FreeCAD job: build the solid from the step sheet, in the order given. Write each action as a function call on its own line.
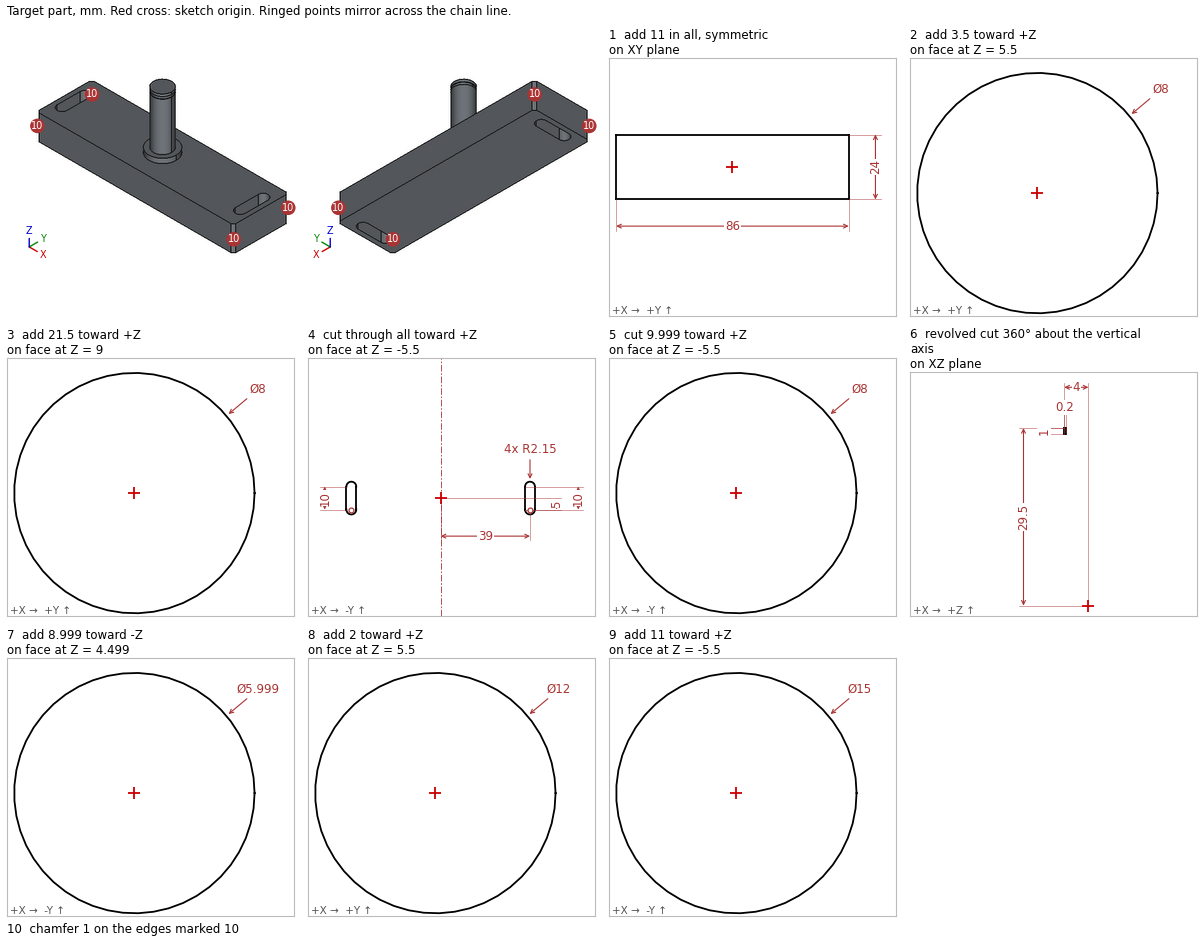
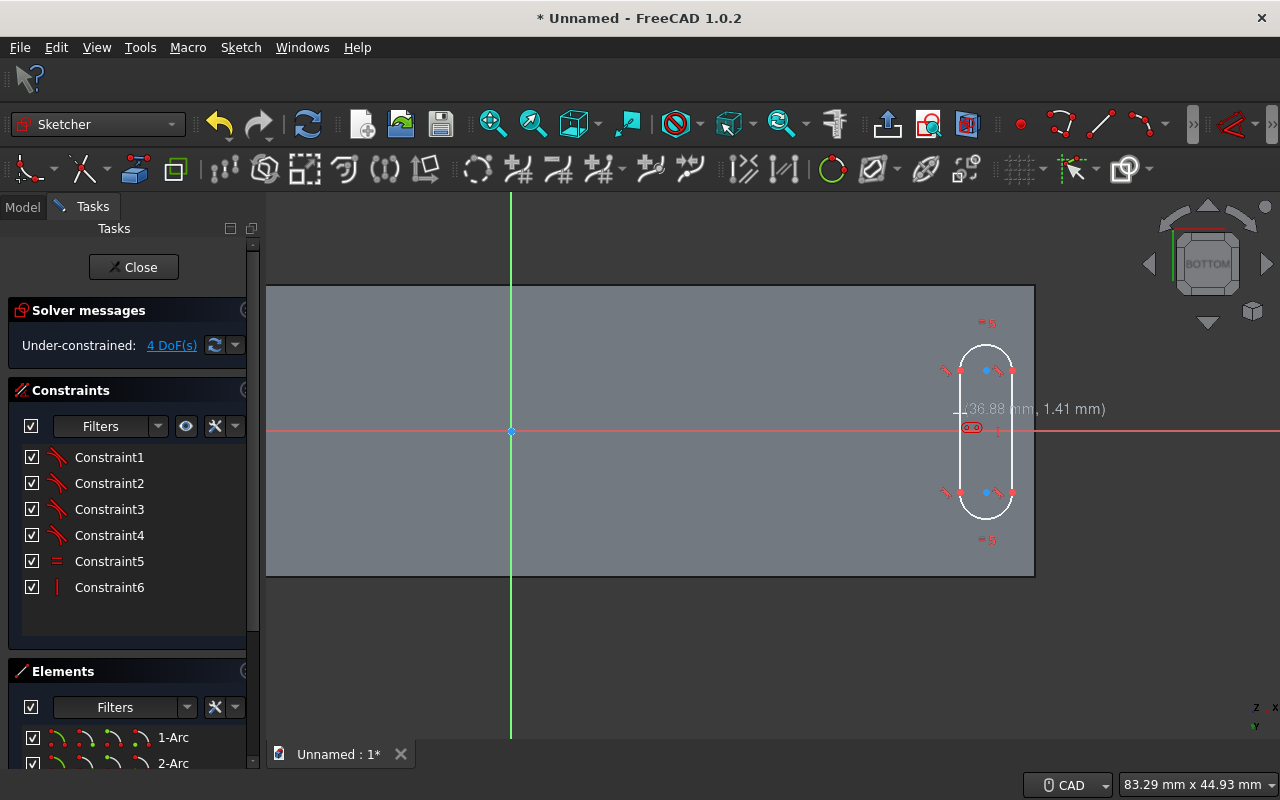
scroll(940, 507, down, 3)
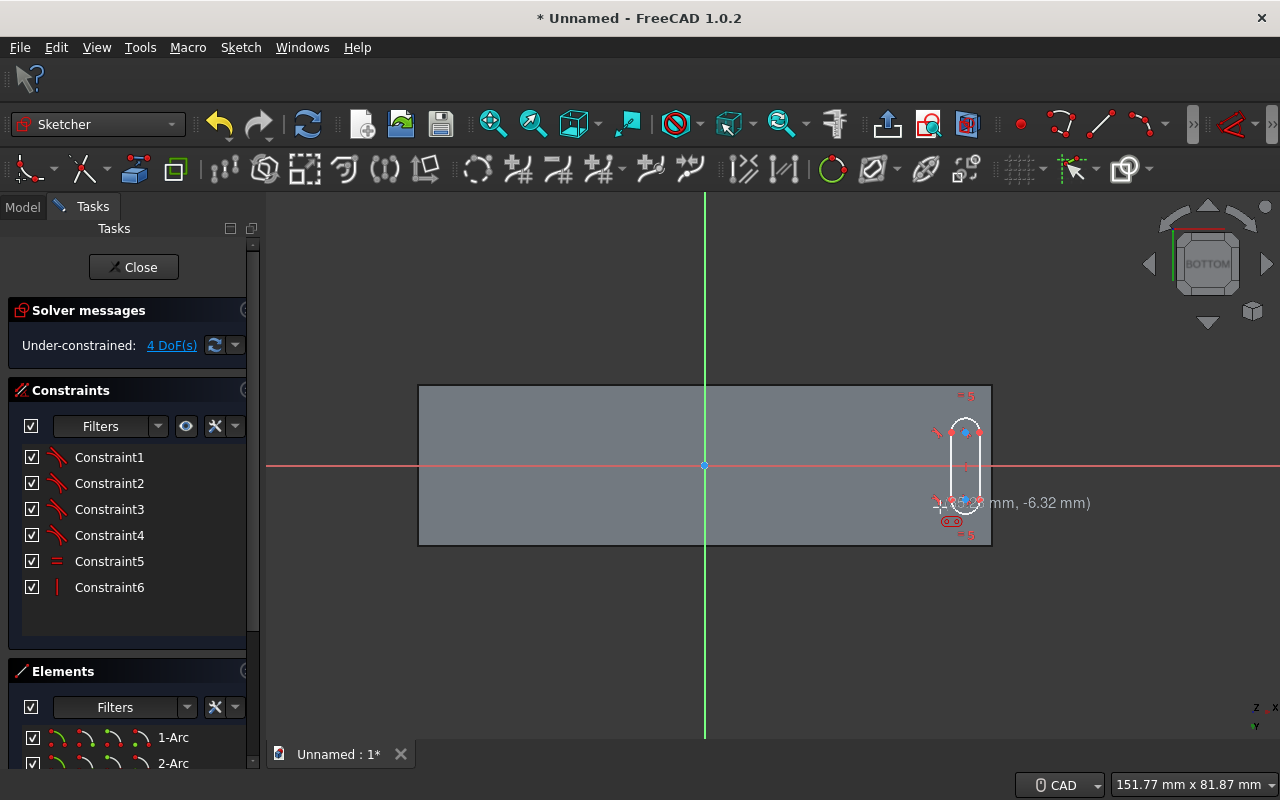
scroll(444, 499, up, 3)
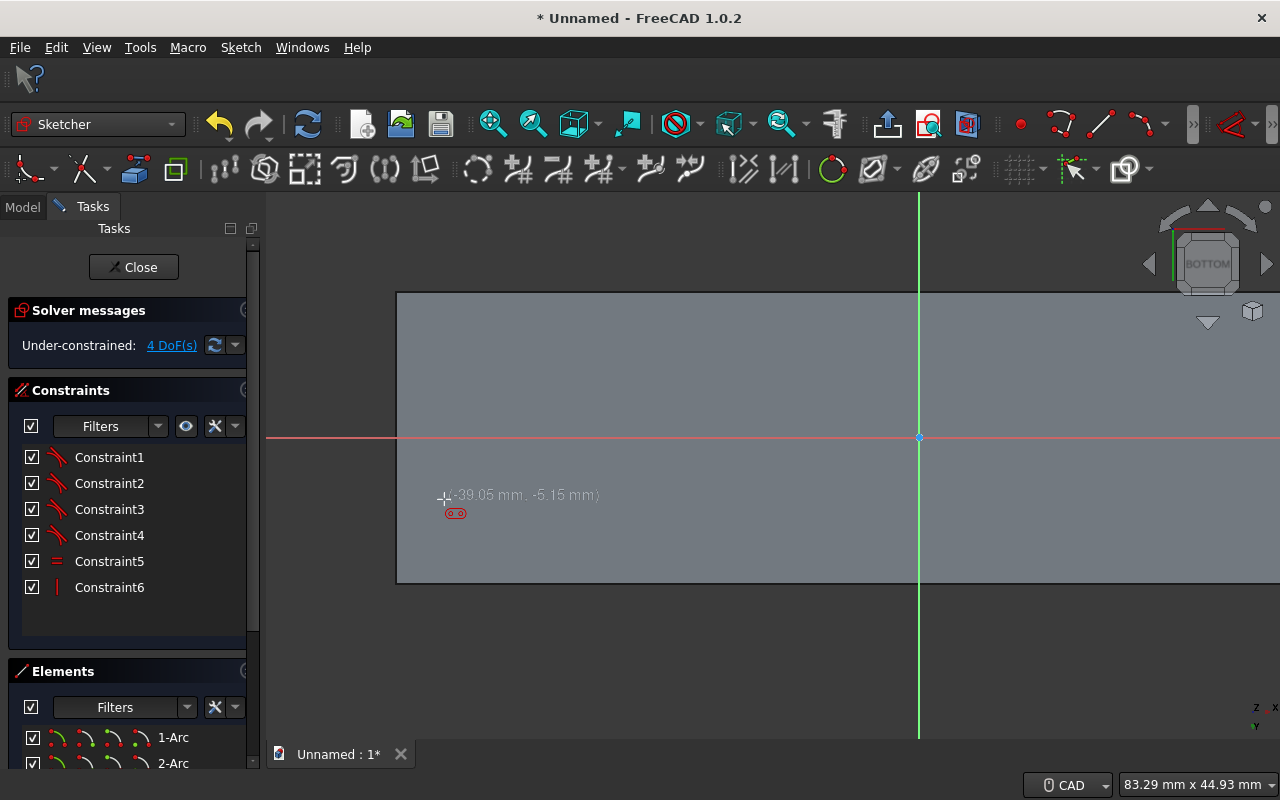
click(444, 499)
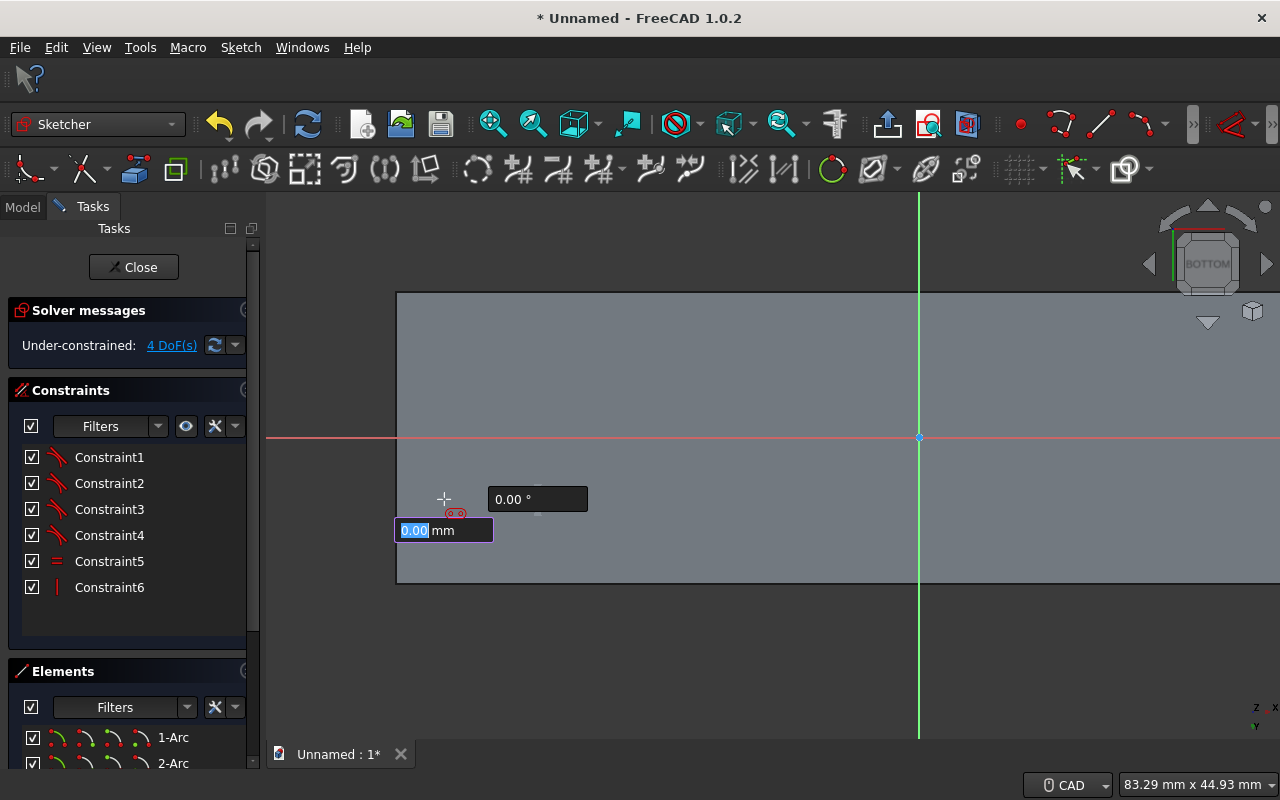
click(444, 377)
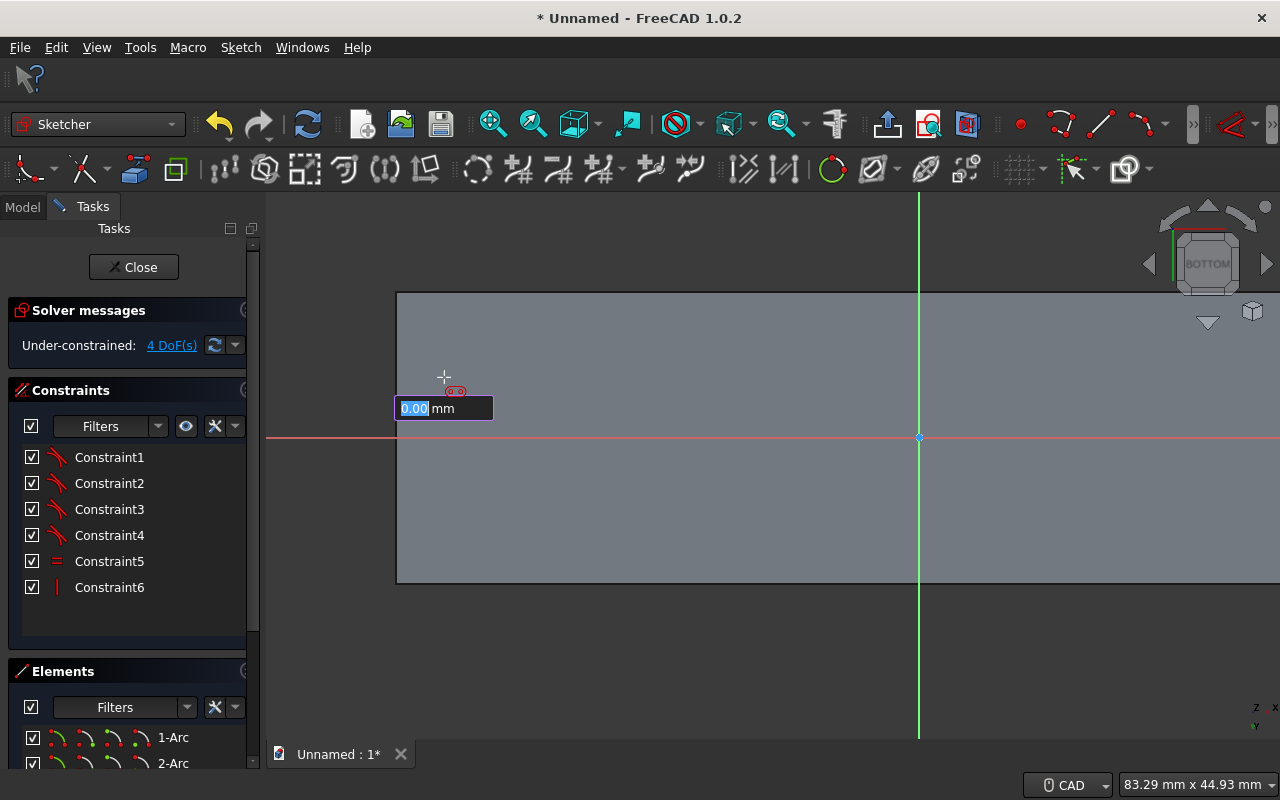
click(471, 456)
key(Escape)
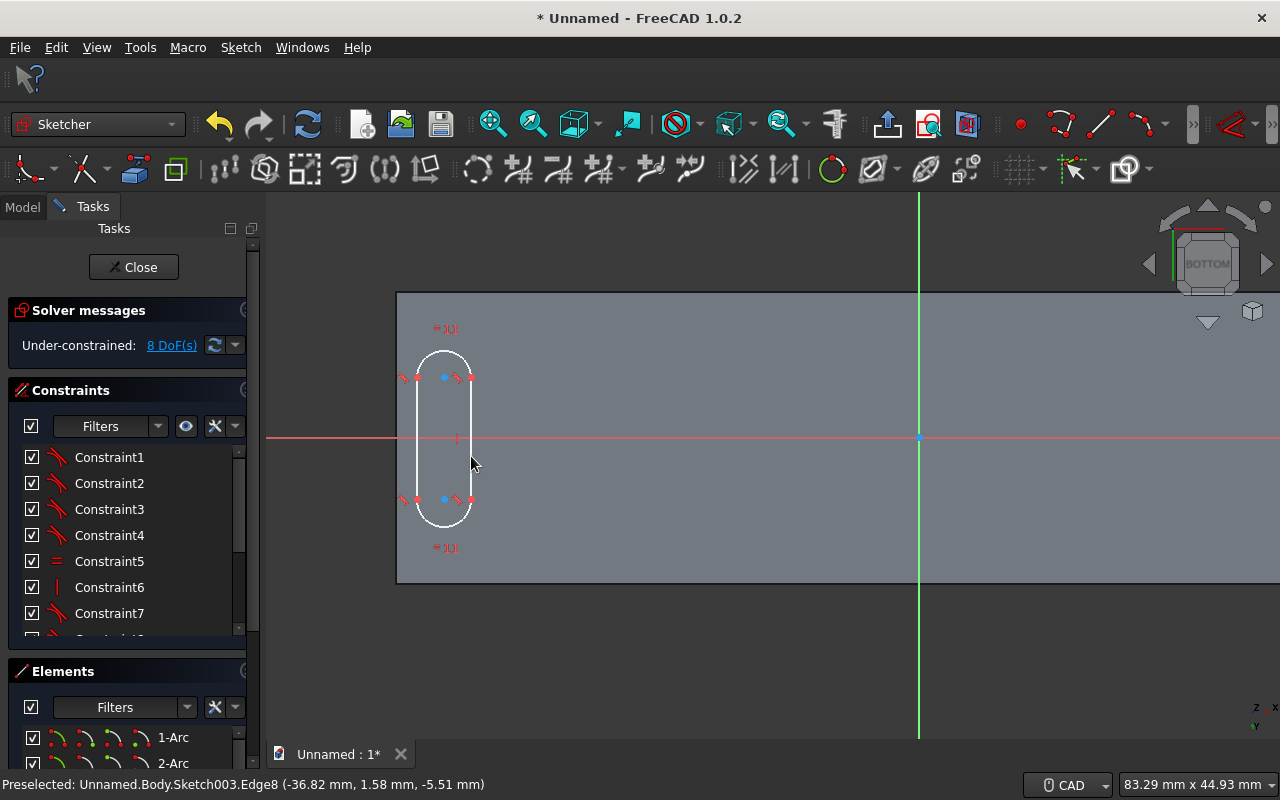
scroll(443, 499, down, 3)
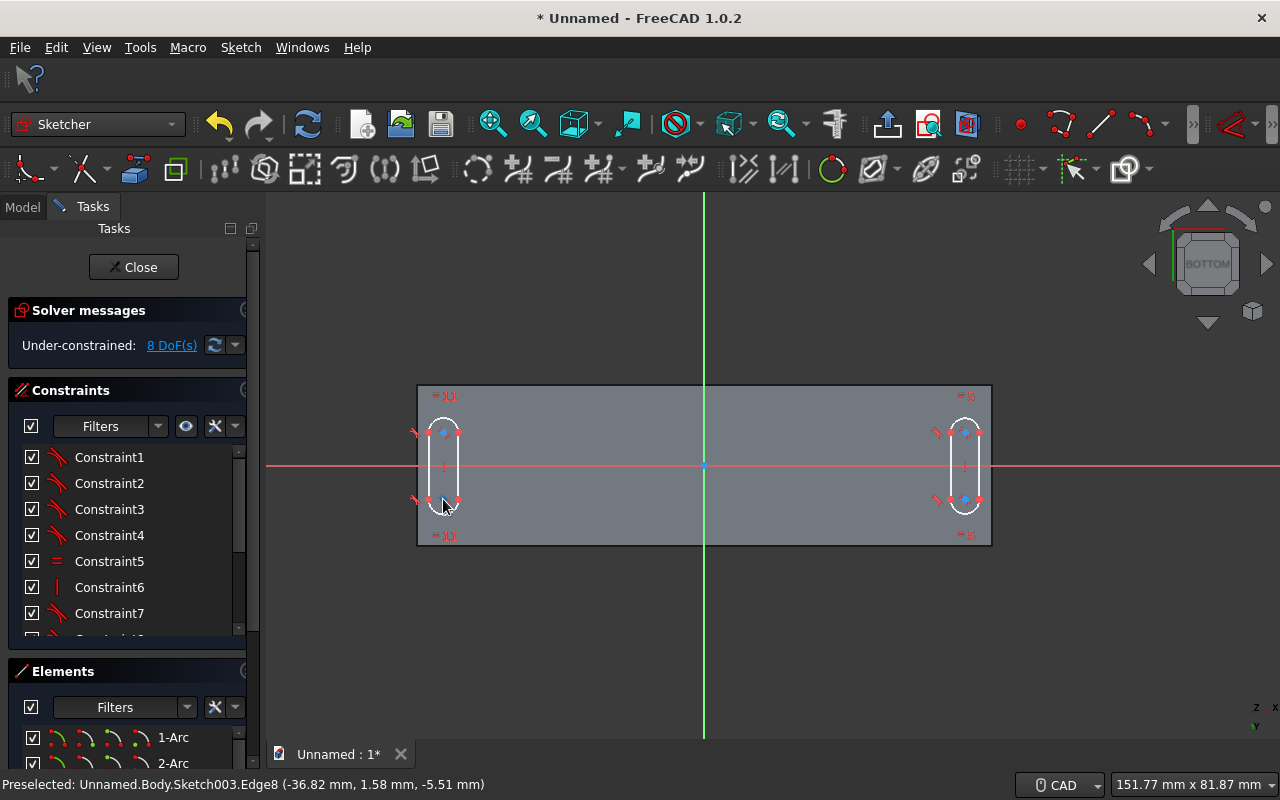
click(957, 511)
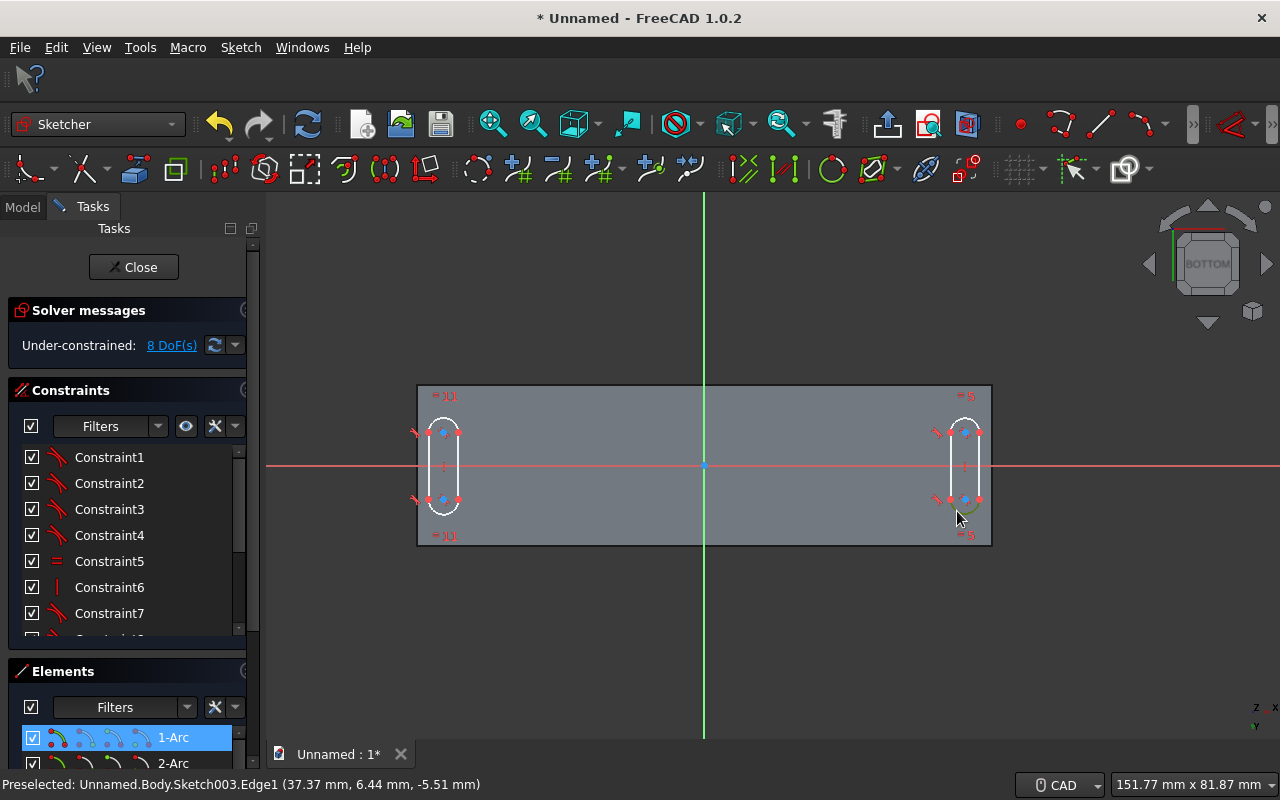
click(435, 512)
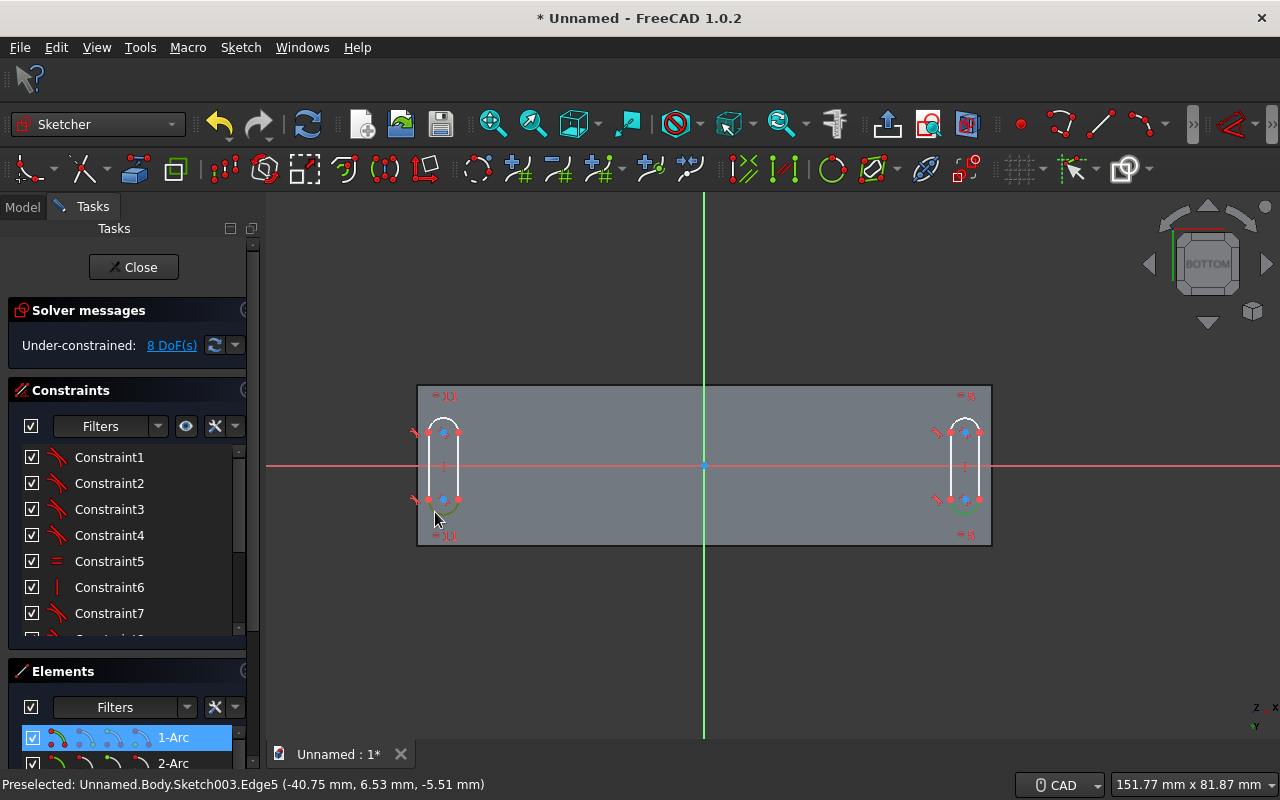
key(e)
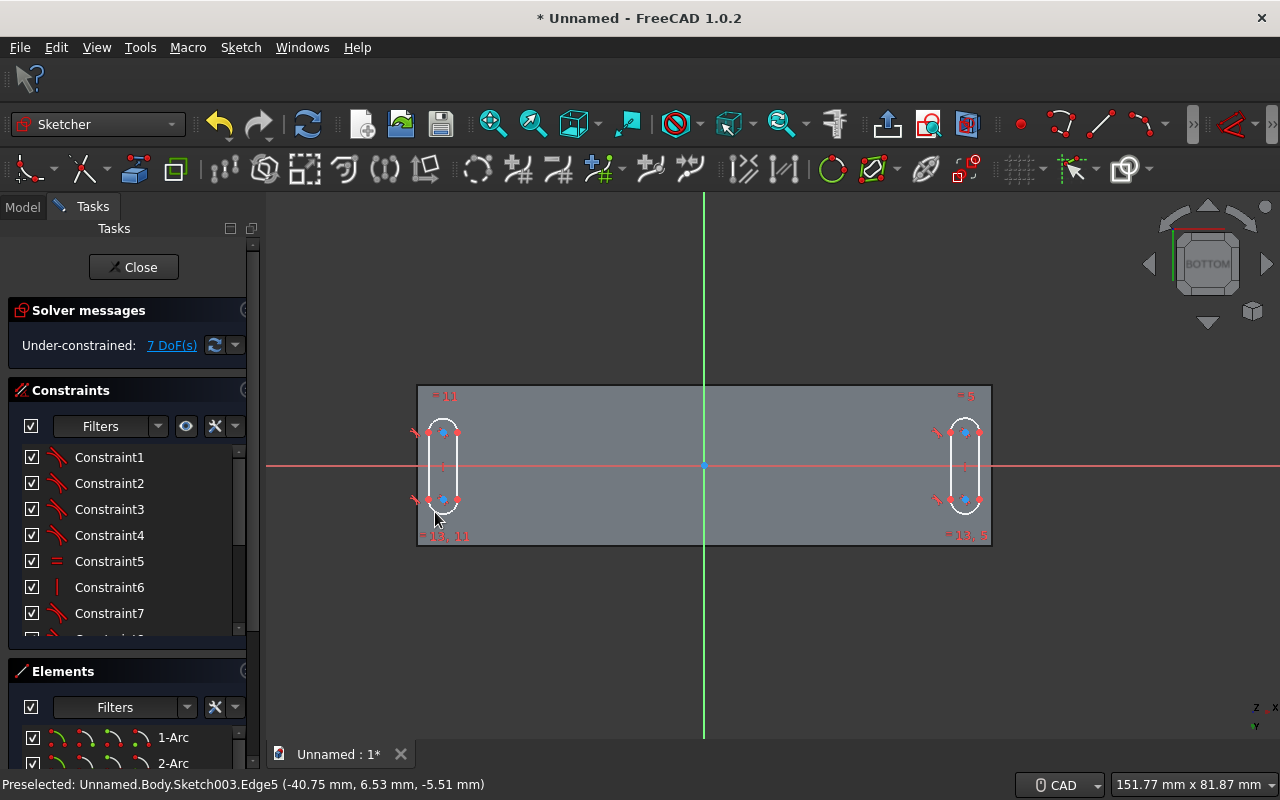
click(965, 500)